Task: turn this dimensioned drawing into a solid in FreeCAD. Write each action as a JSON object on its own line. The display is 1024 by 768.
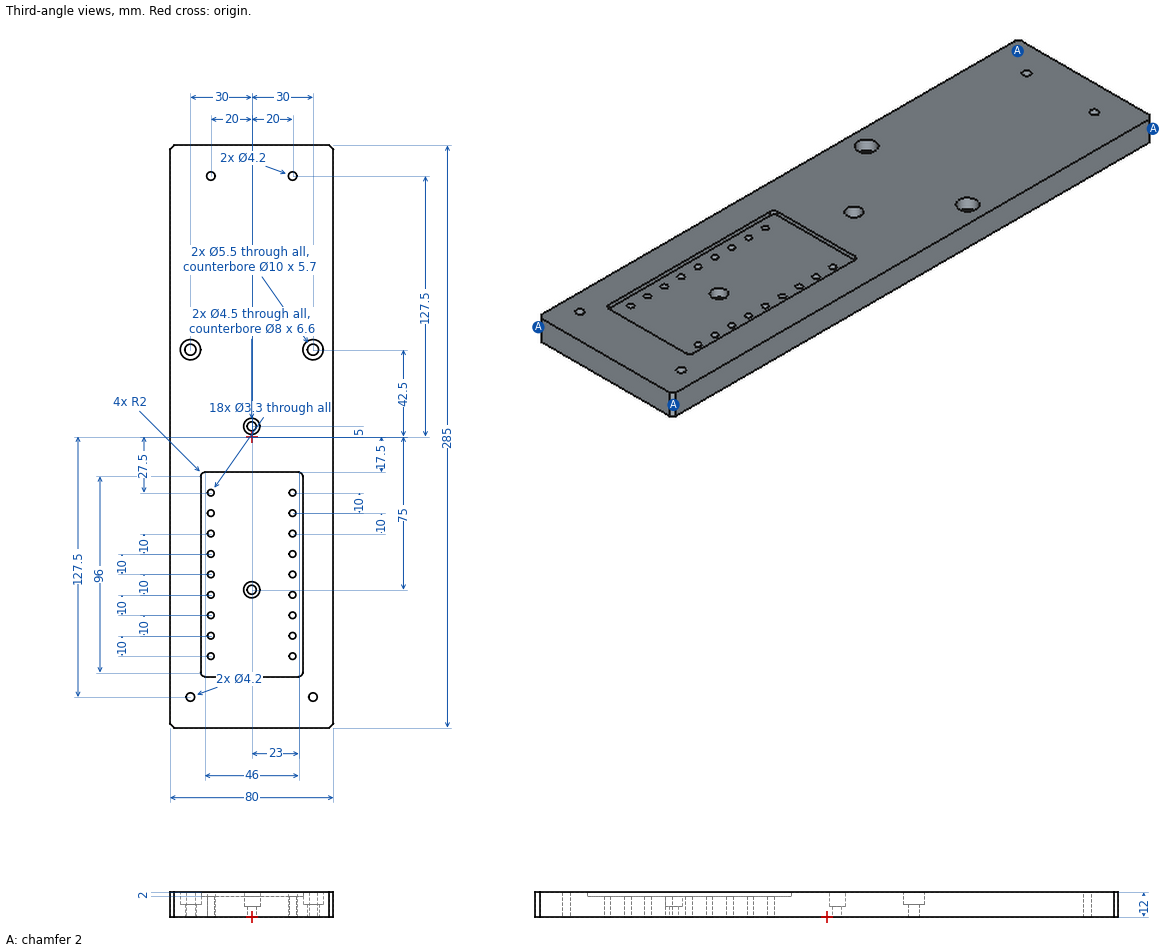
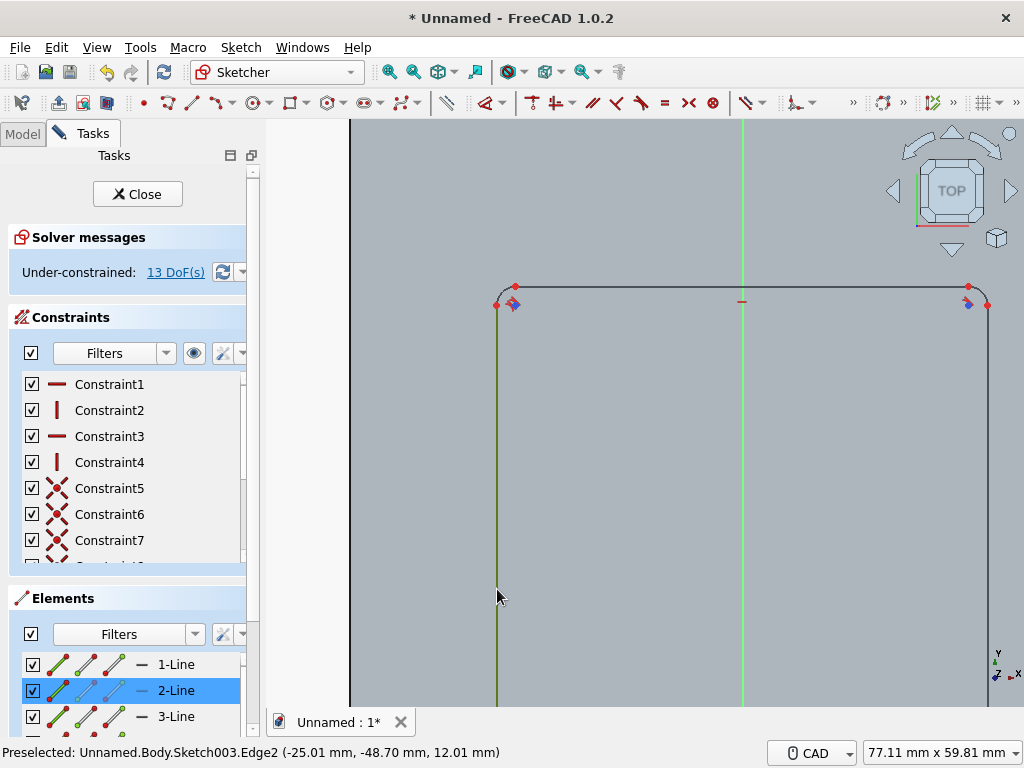
{"action": "scroll", "coordinate": [505, 294], "scroll_direction": "down", "scroll_amount": 6}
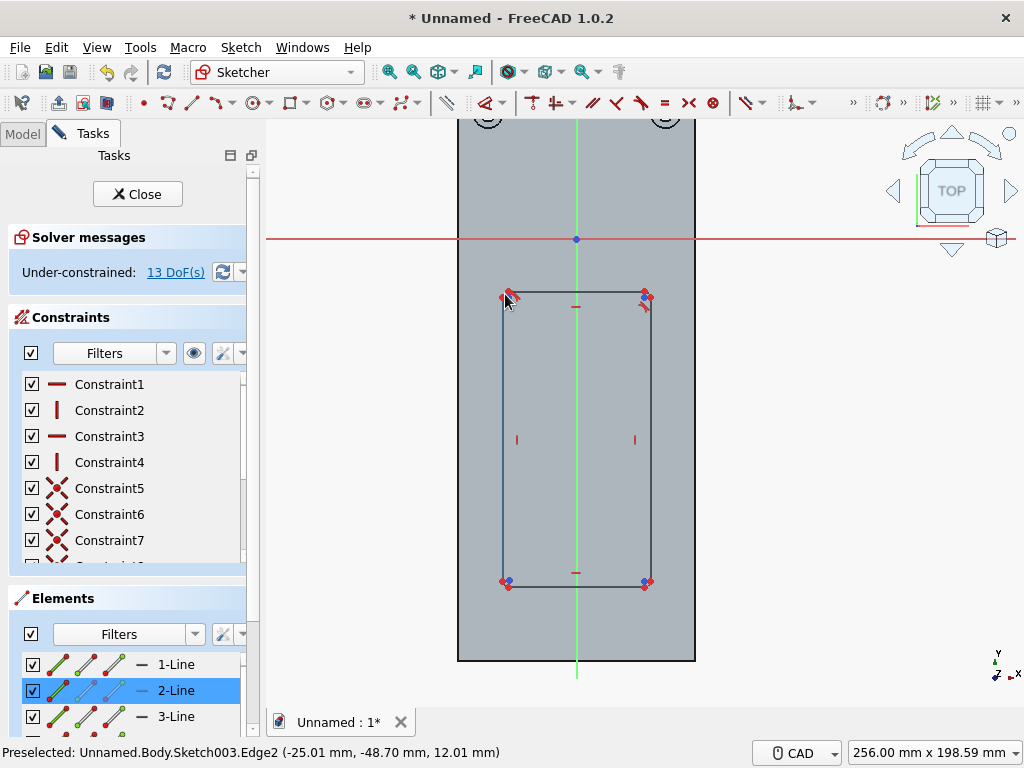
{"action": "scroll", "coordinate": [505, 586], "scroll_direction": "up", "scroll_amount": 6}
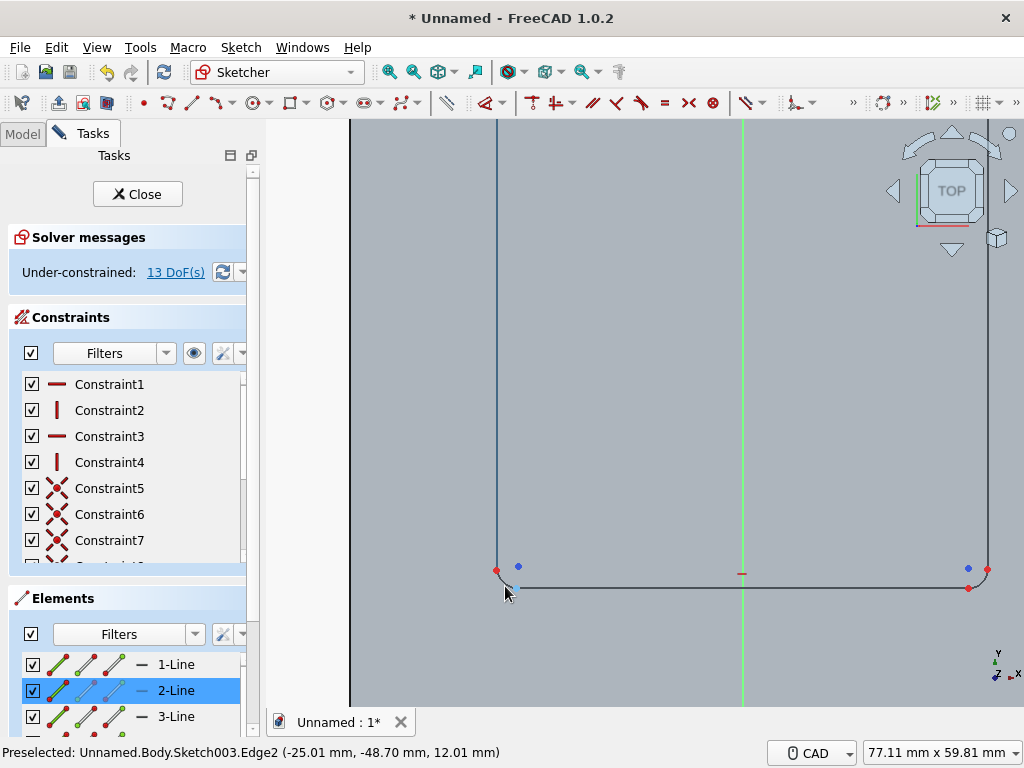
{"action": "left_click", "coordinate": [504, 583]}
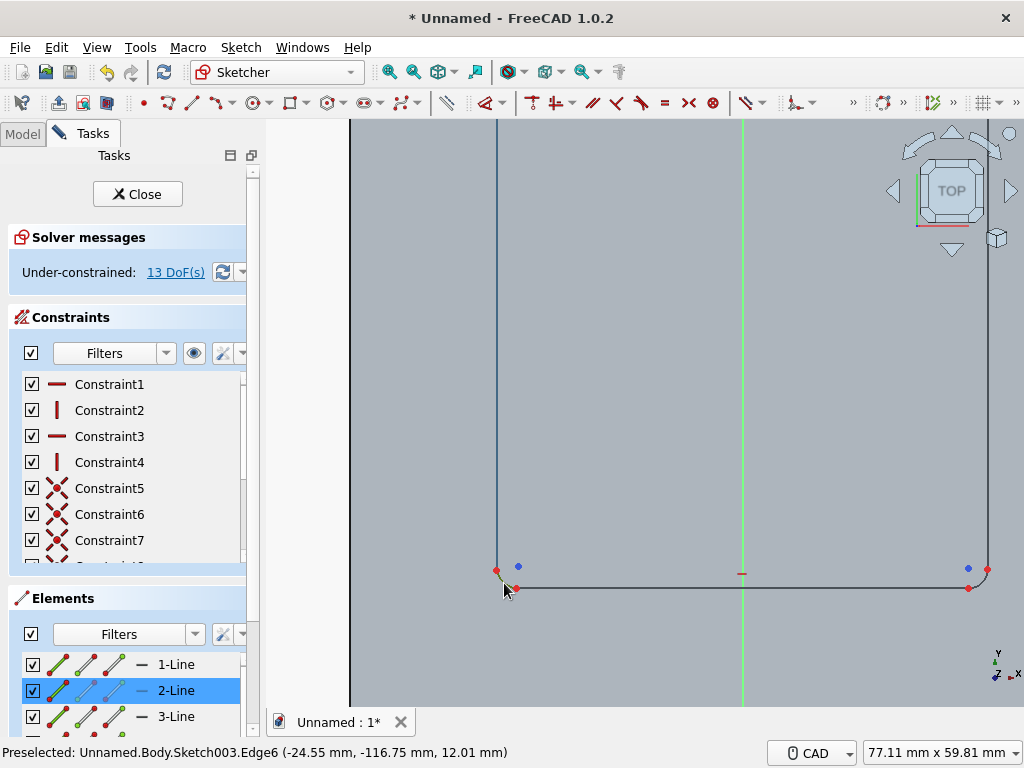
{"action": "key", "text": "t"}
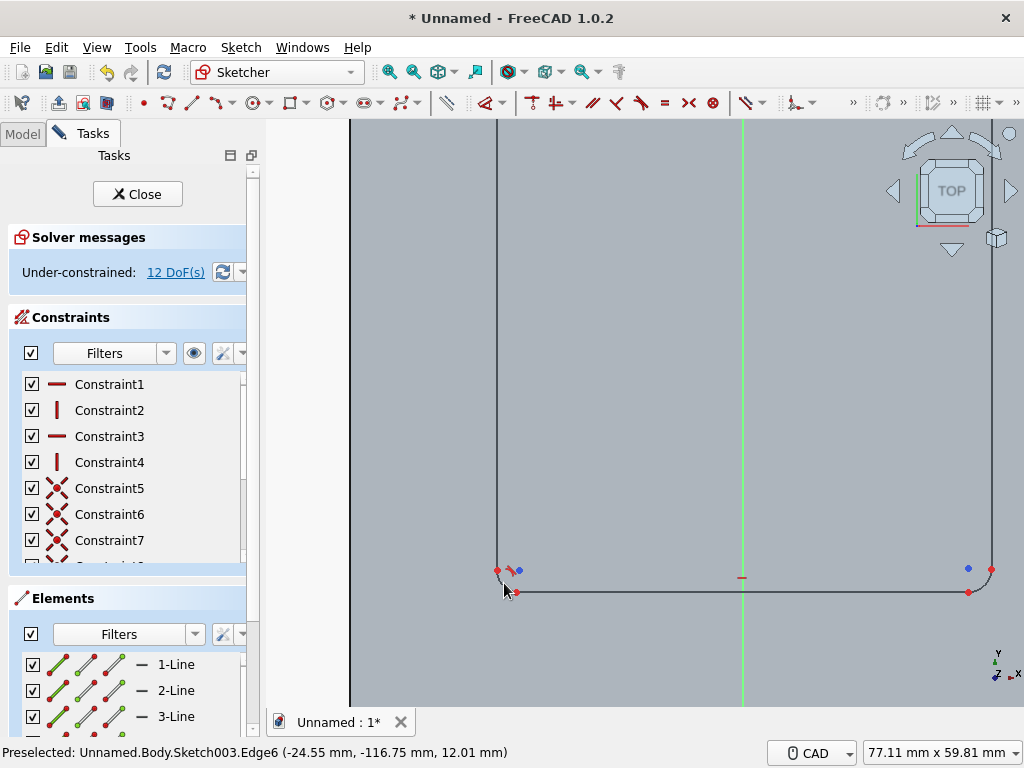
{"action": "left_click", "coordinate": [652, 592]}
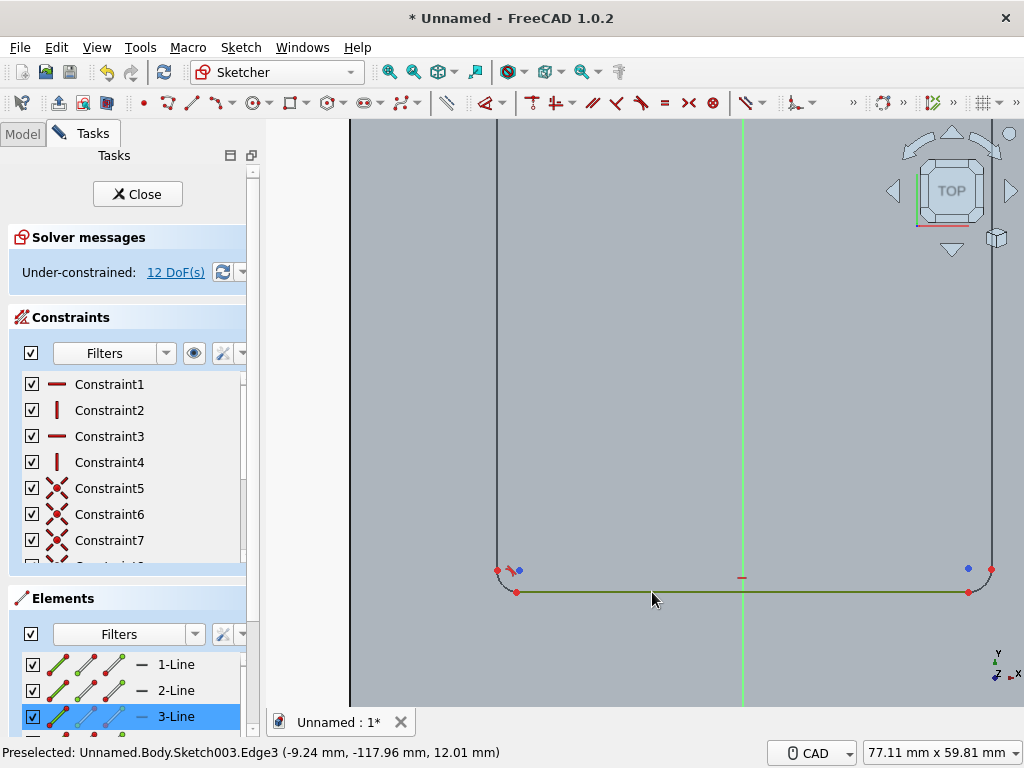
{"action": "scroll", "coordinate": [499, 580], "scroll_direction": "up", "scroll_amount": 2}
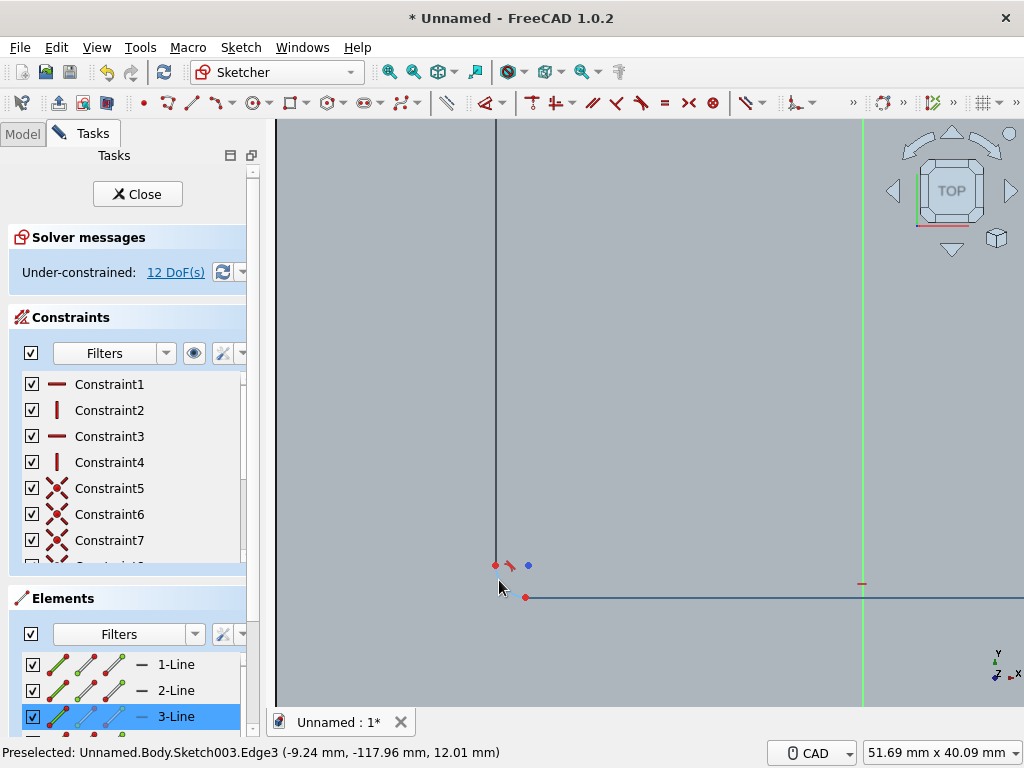
{"action": "left_click", "coordinate": [499, 579]}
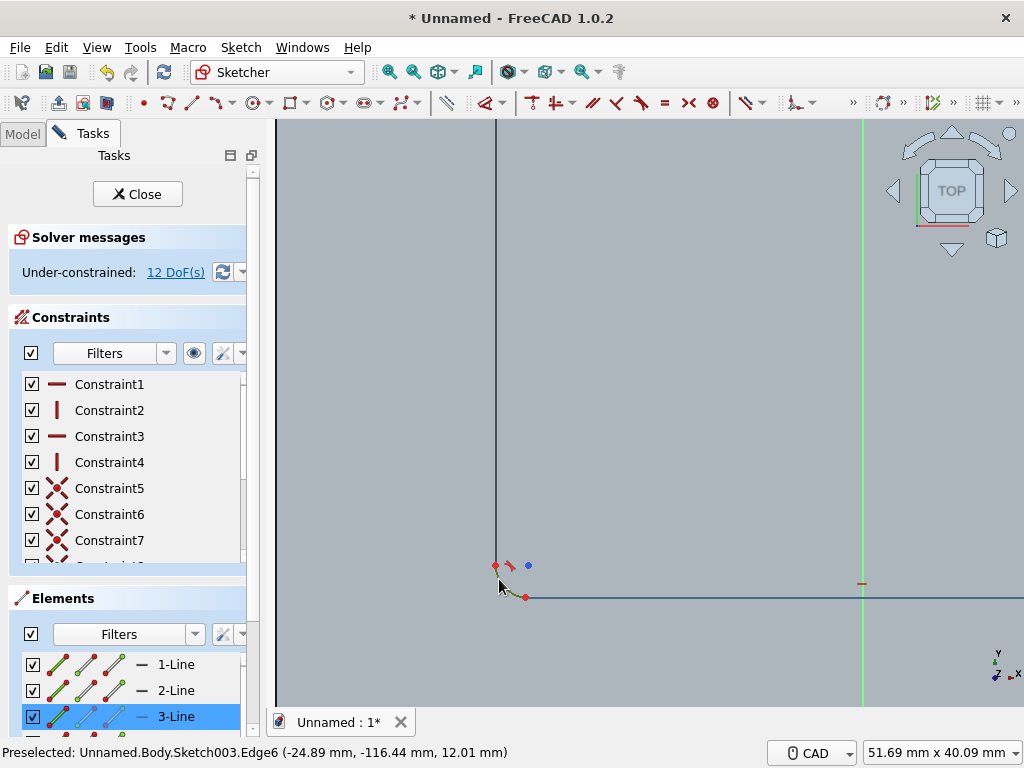
{"action": "left_click", "coordinate": [642, 104]}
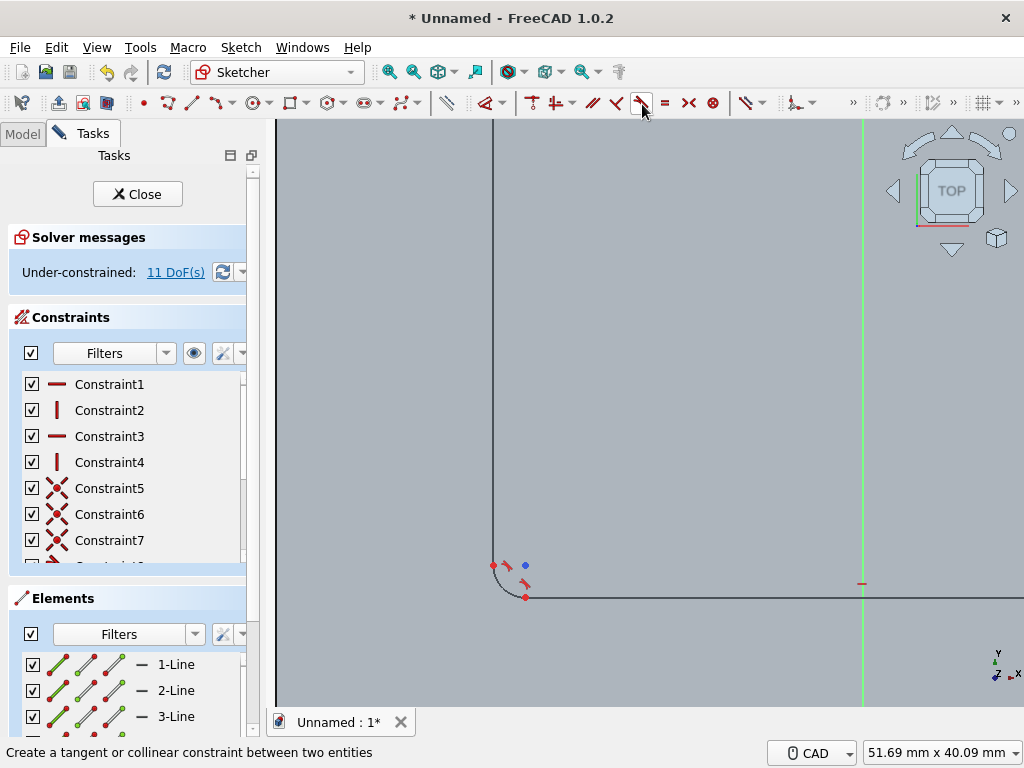
{"action": "scroll", "coordinate": [504, 586], "scroll_direction": "down", "scroll_amount": 8}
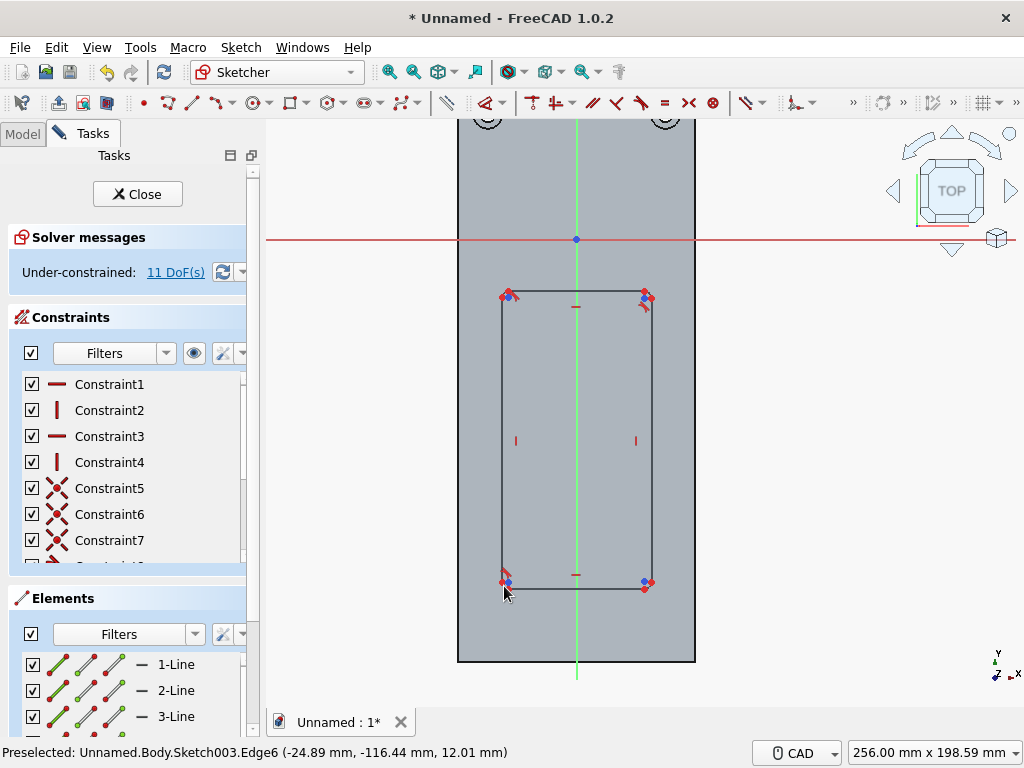
{"action": "left_click", "coordinate": [549, 589]}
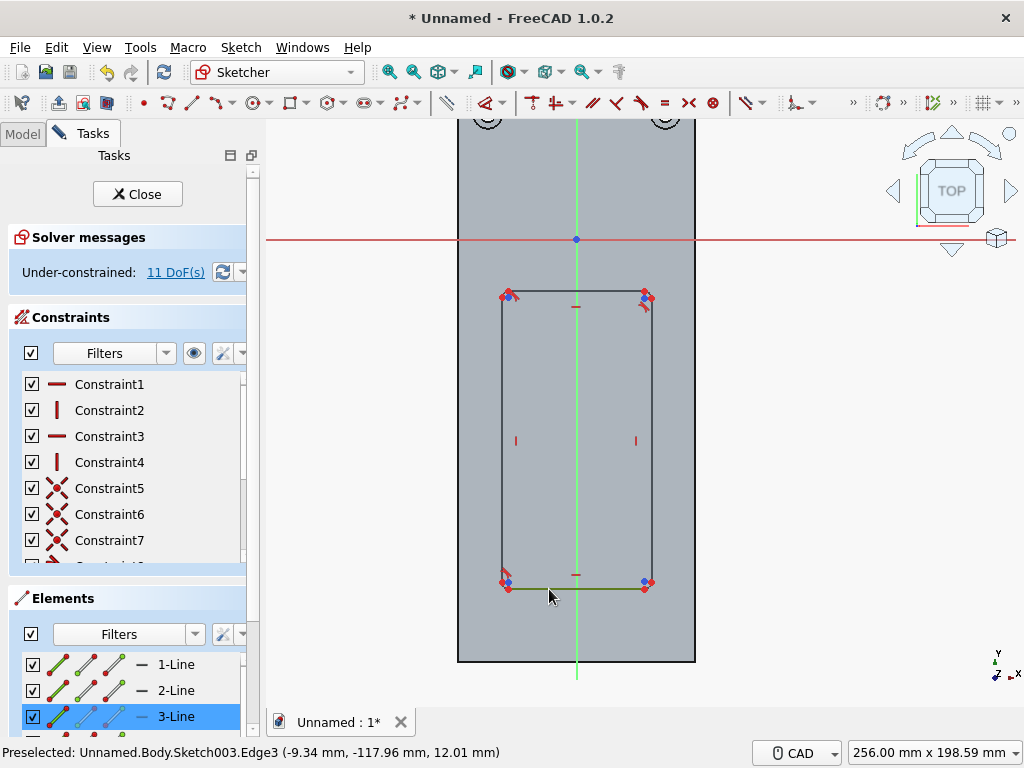
{"action": "scroll", "coordinate": [650, 587], "scroll_direction": "up", "scroll_amount": 5}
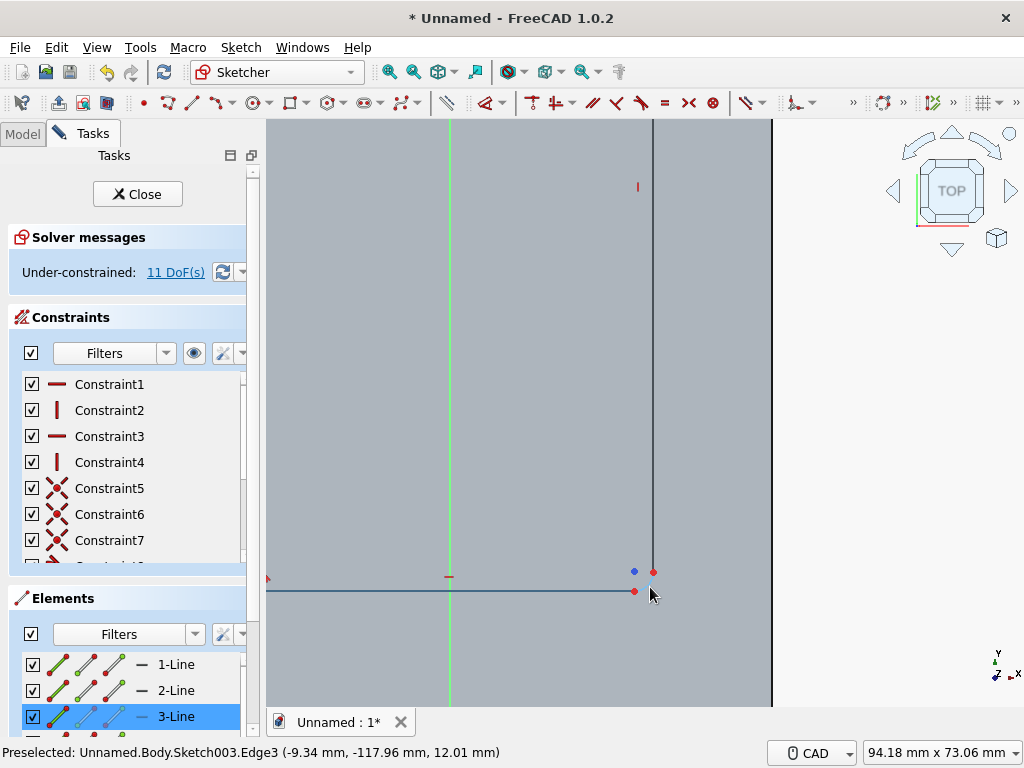
{"action": "left_click", "coordinate": [648, 586]}